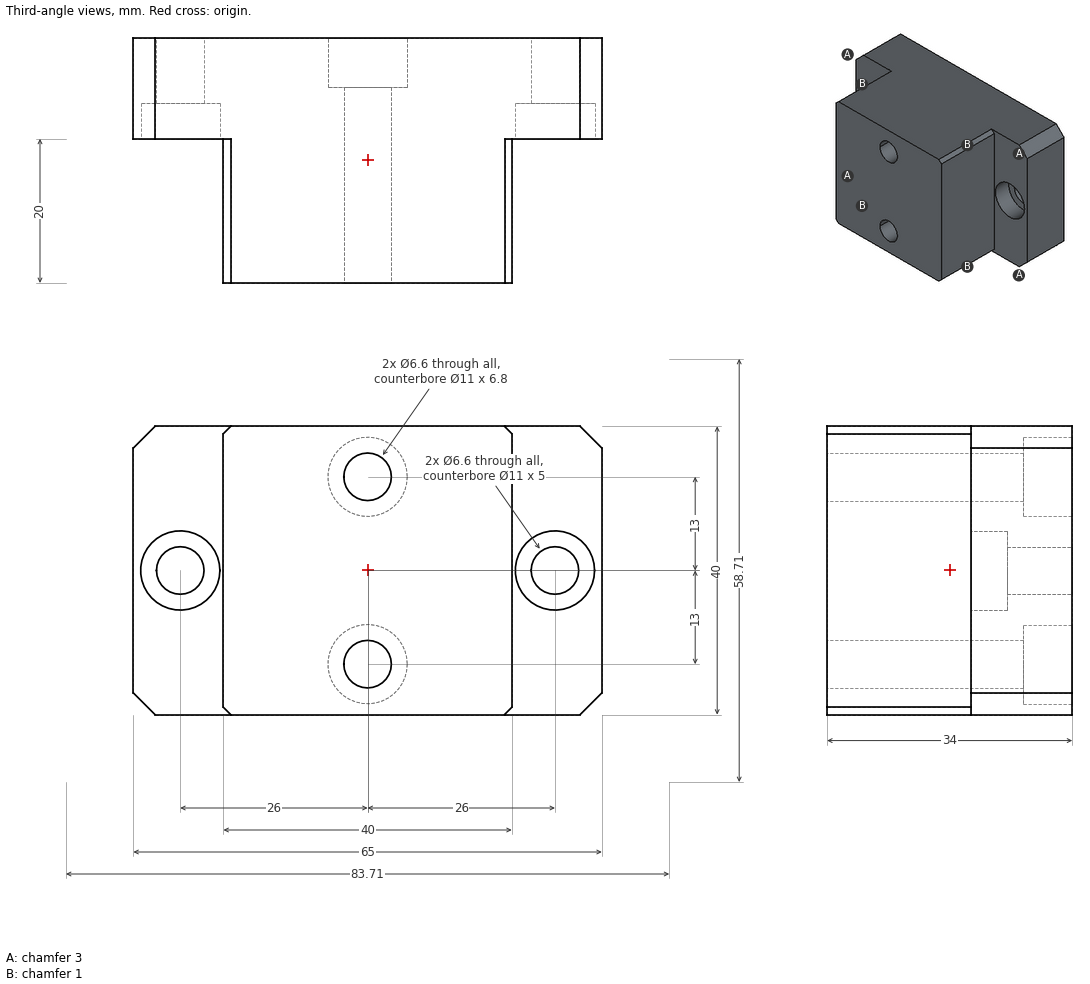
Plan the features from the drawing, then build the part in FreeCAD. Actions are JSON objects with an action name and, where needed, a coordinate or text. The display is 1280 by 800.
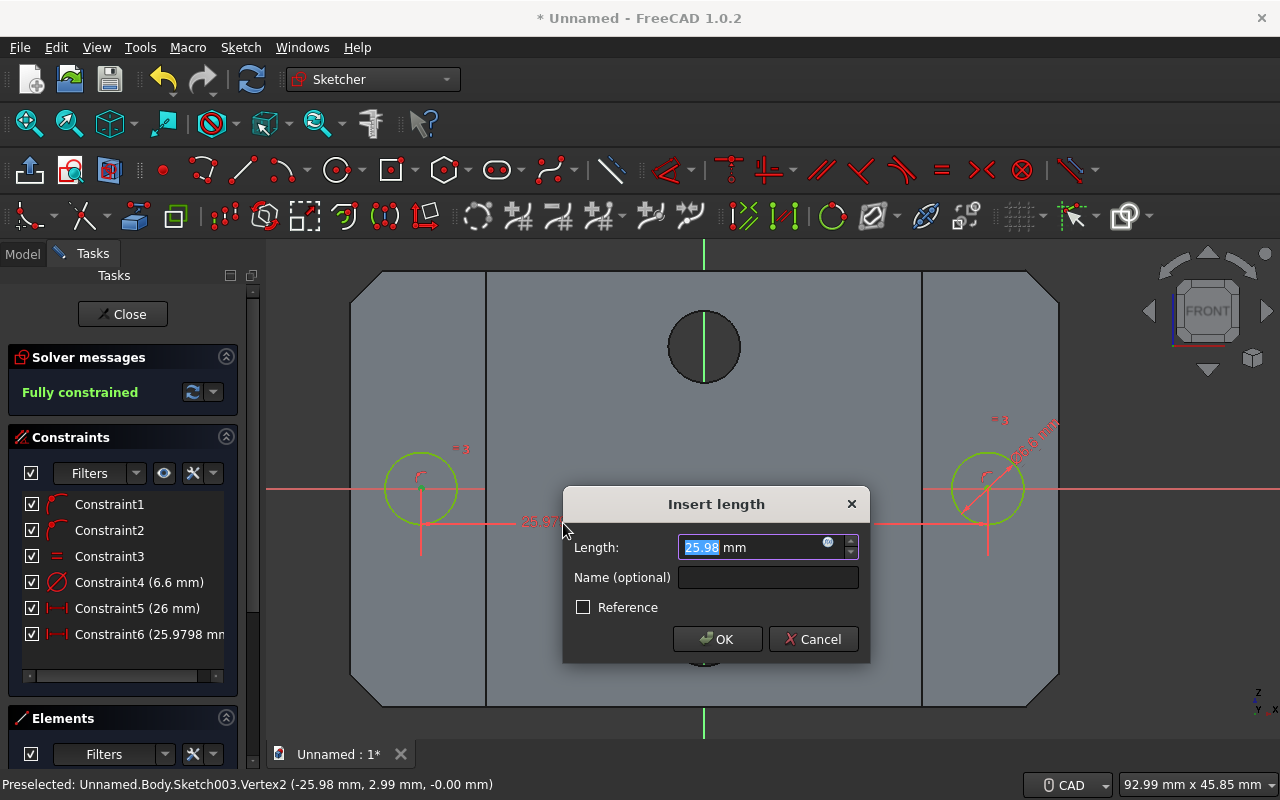
{"action": "type", "text": "26"}
{"action": "key", "text": "Return"}
{"action": "key", "text": "Escape"}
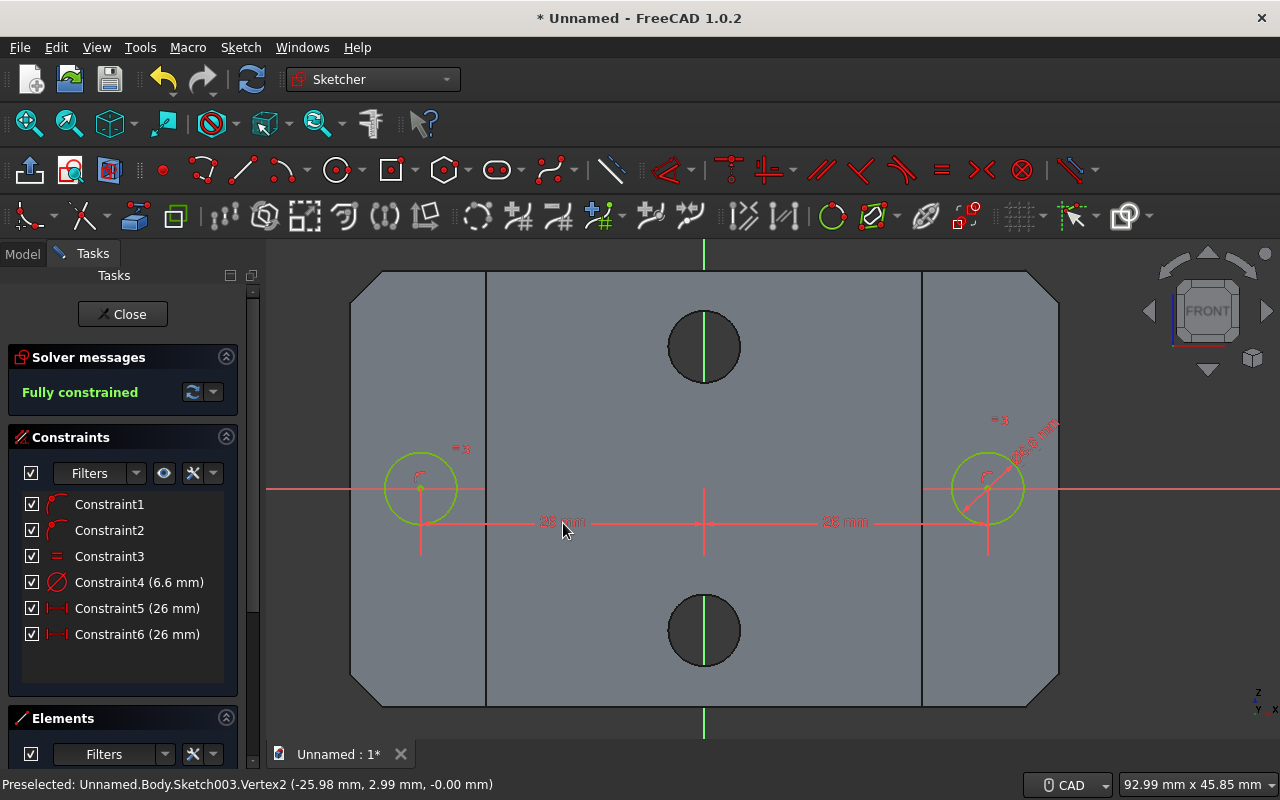
{"action": "left_click", "coordinate": [123, 314]}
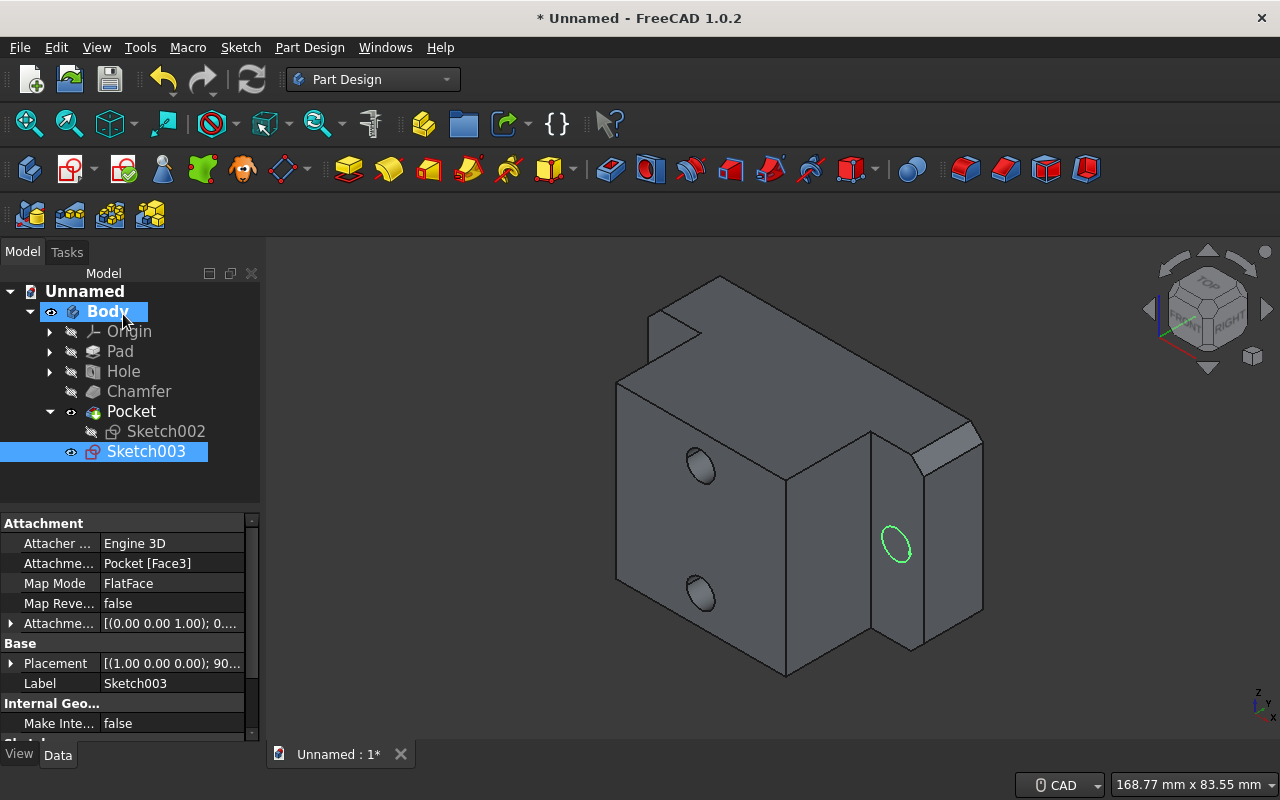
{"action": "left_click", "coordinate": [652, 170]}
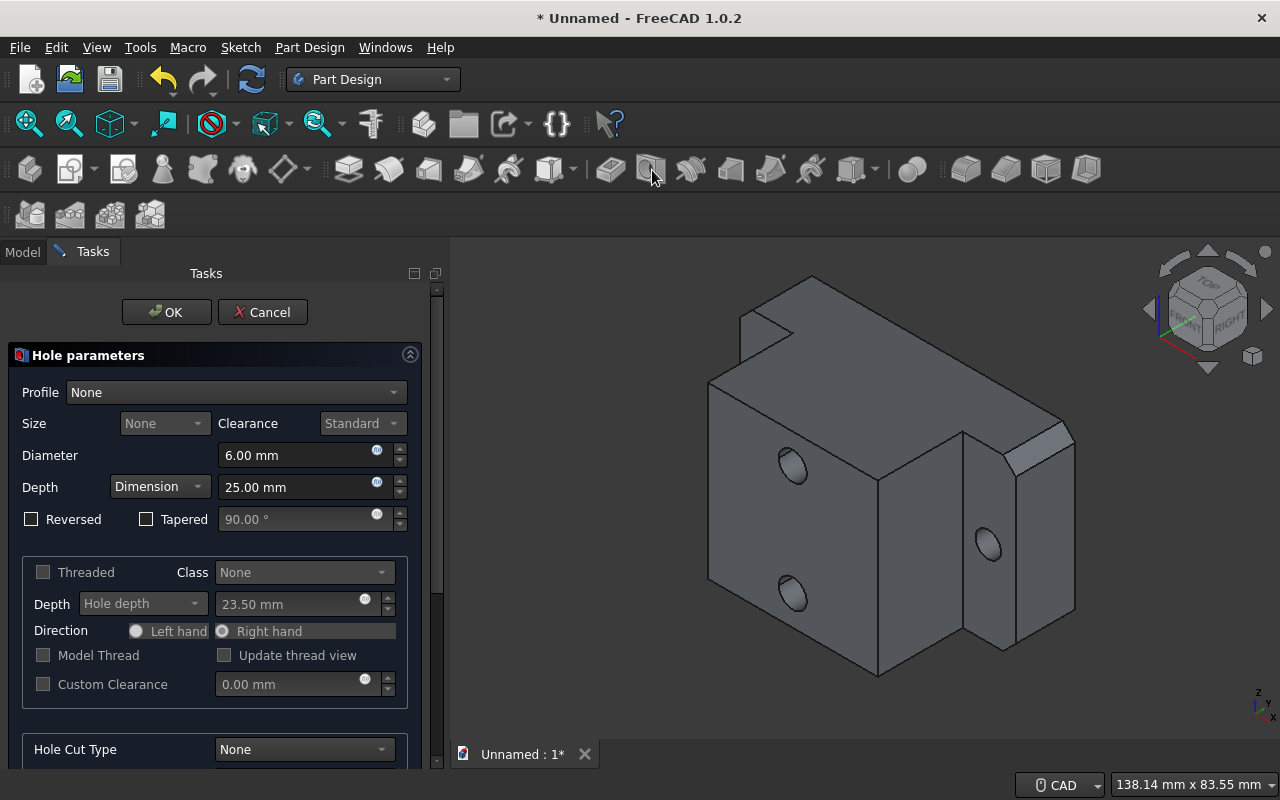
{"action": "triple_click", "coordinate": [305, 455]}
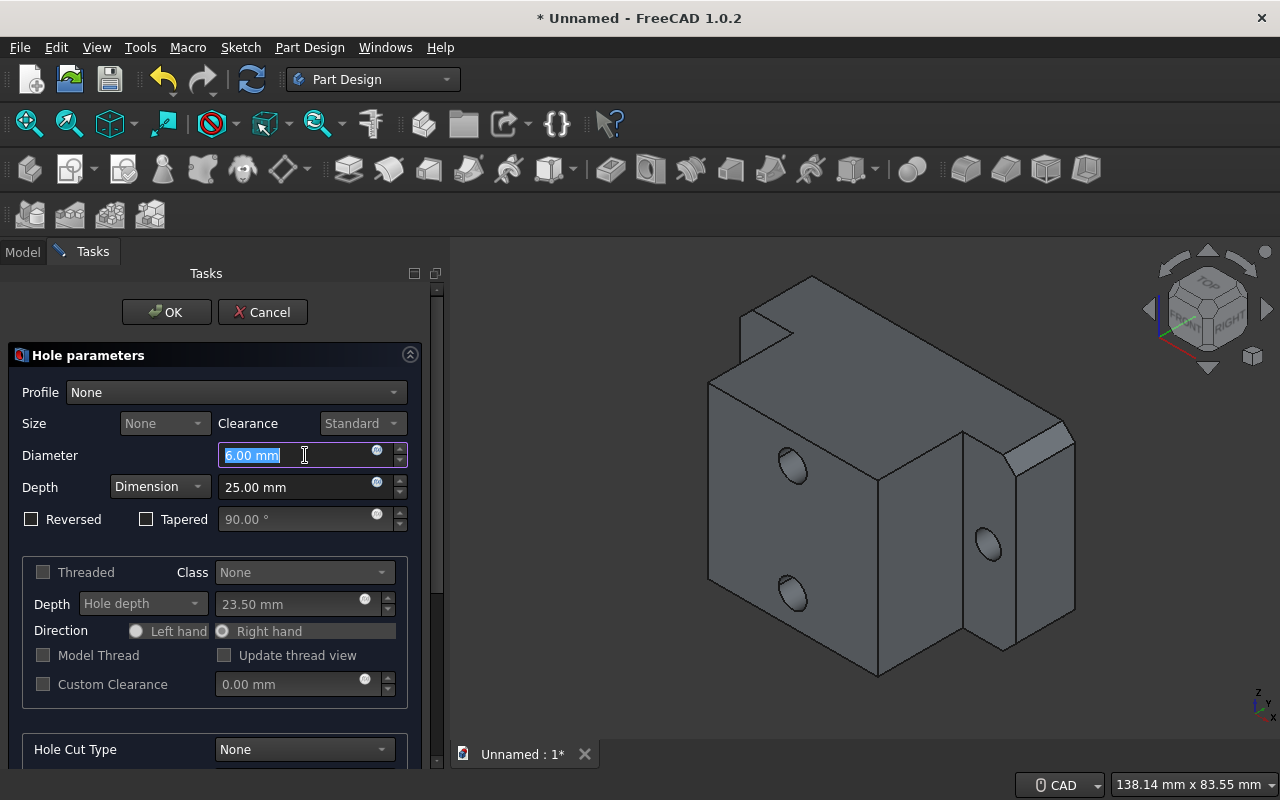
{"action": "type", "text": "6.6"}
{"action": "key", "text": "Tab"}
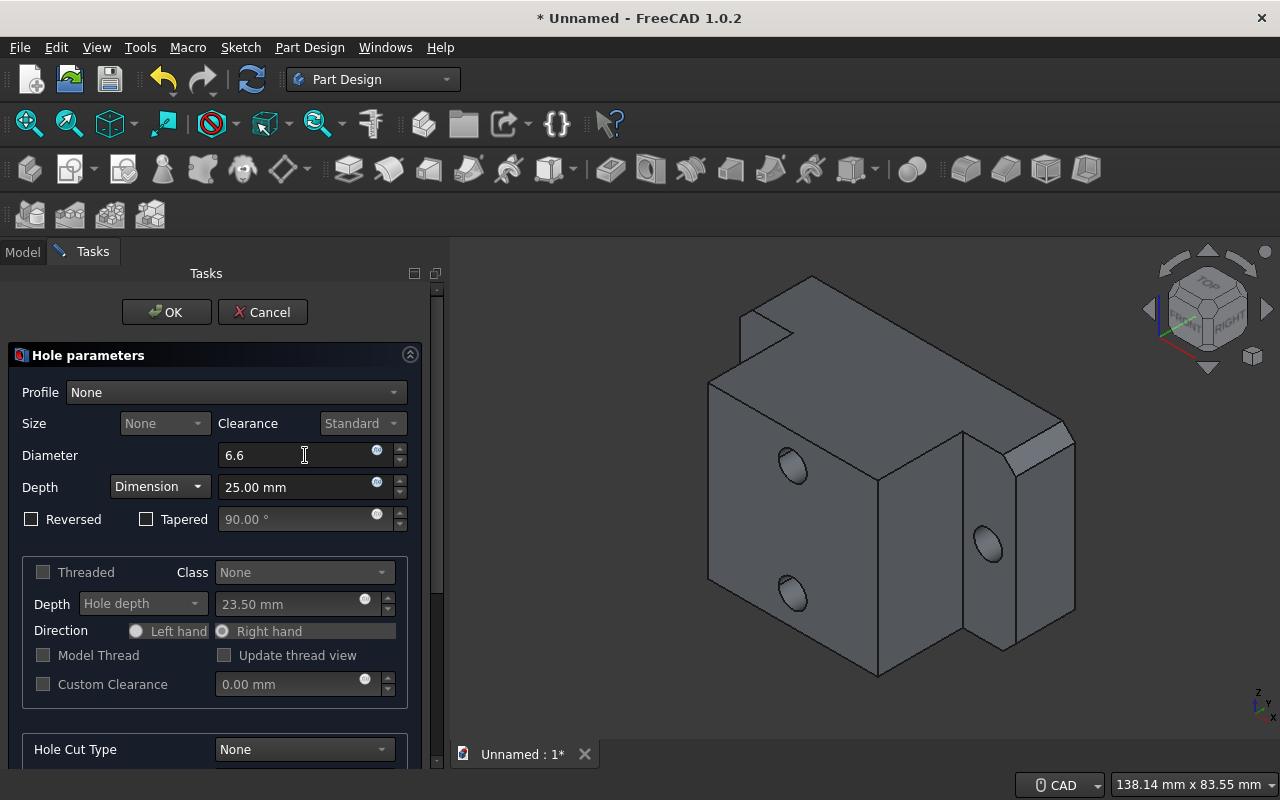
{"action": "left_click", "coordinate": [161, 486]}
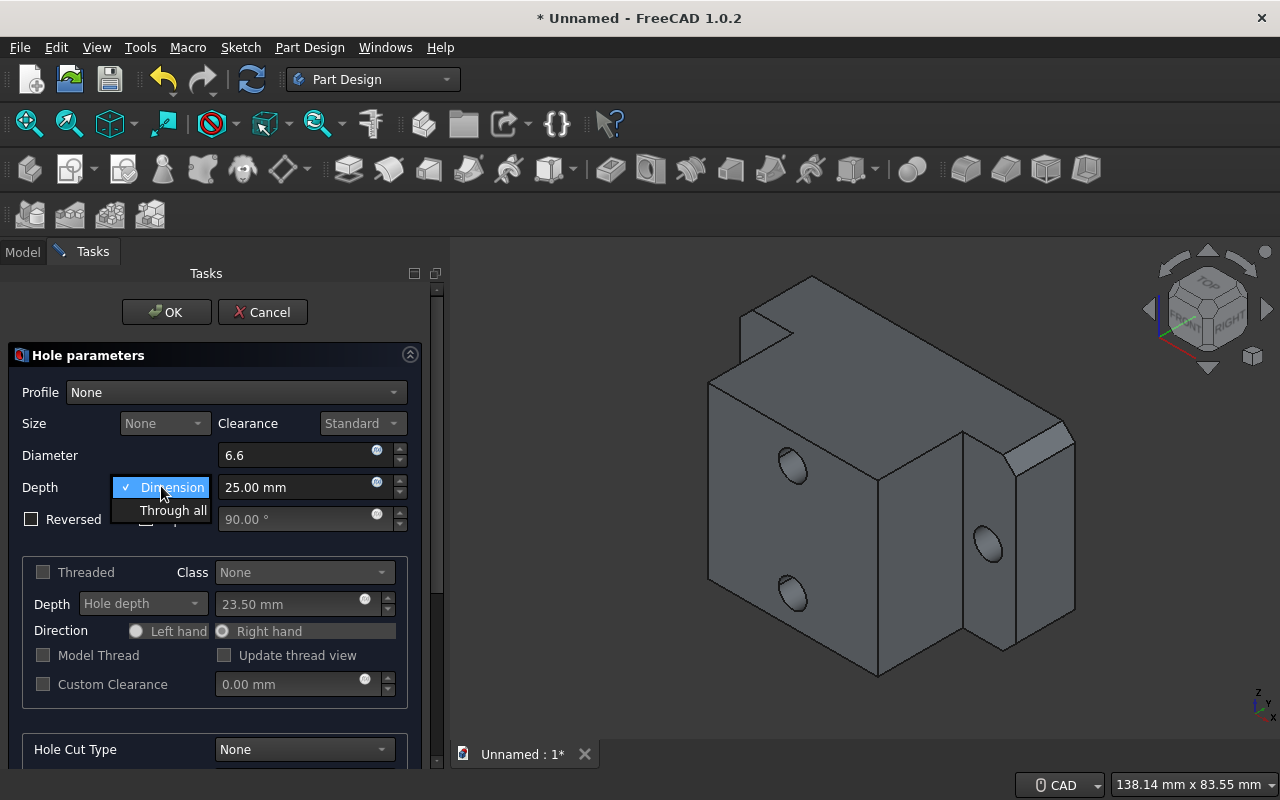
{"action": "left_click", "coordinate": [160, 510]}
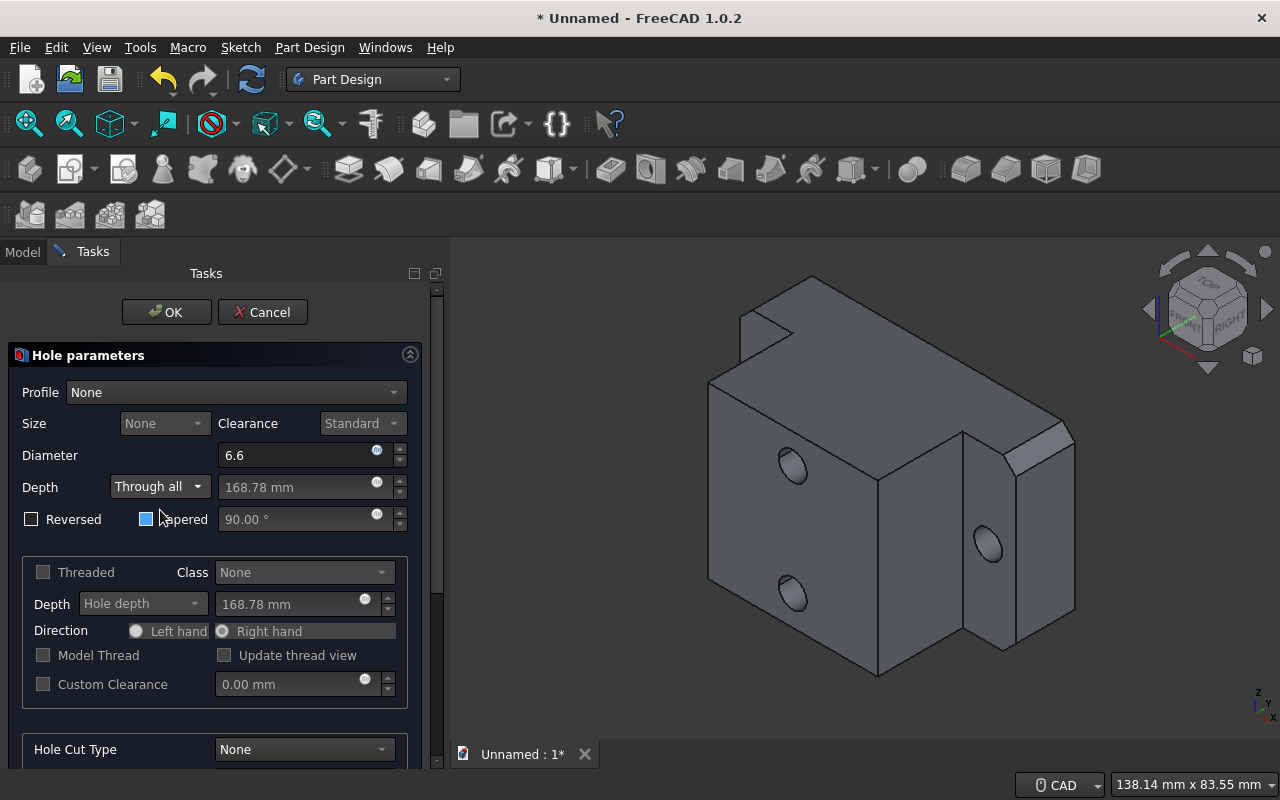
{"action": "left_click", "coordinate": [306, 750]}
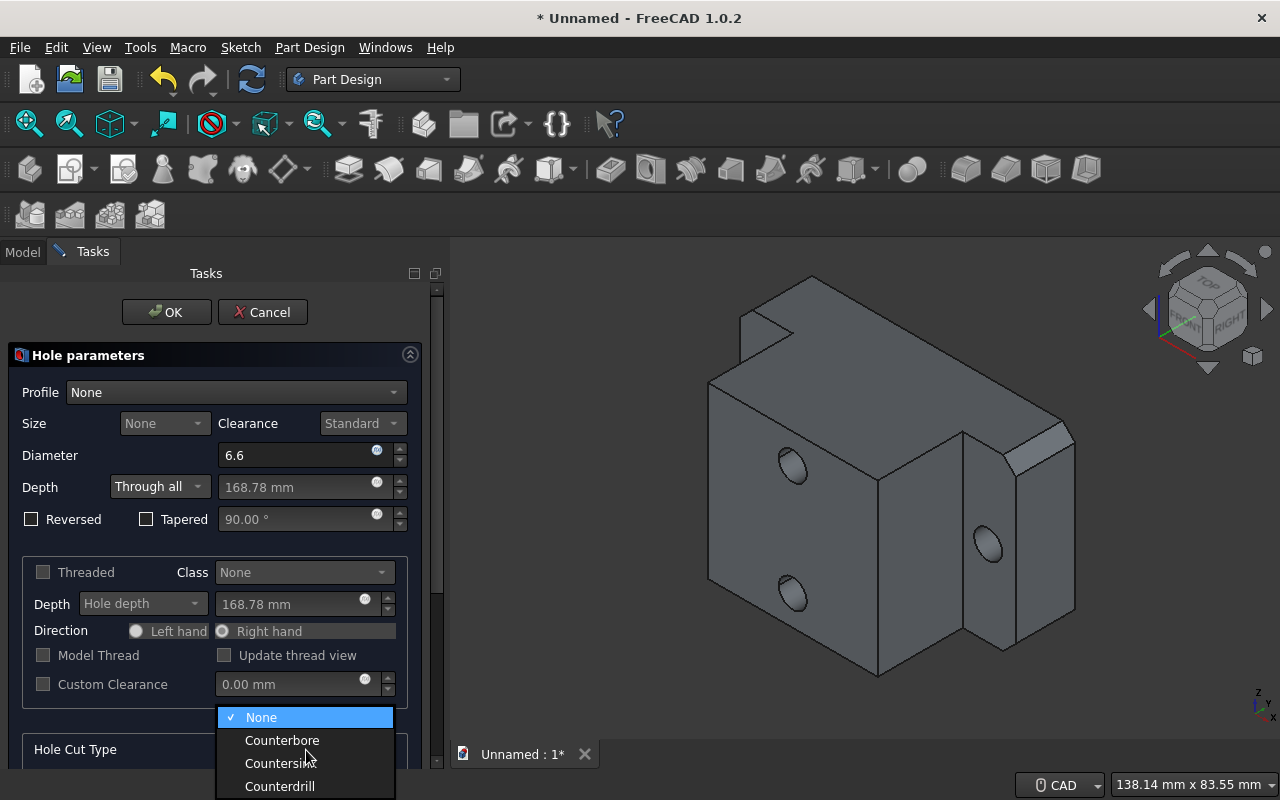
{"action": "left_click", "coordinate": [304, 740]}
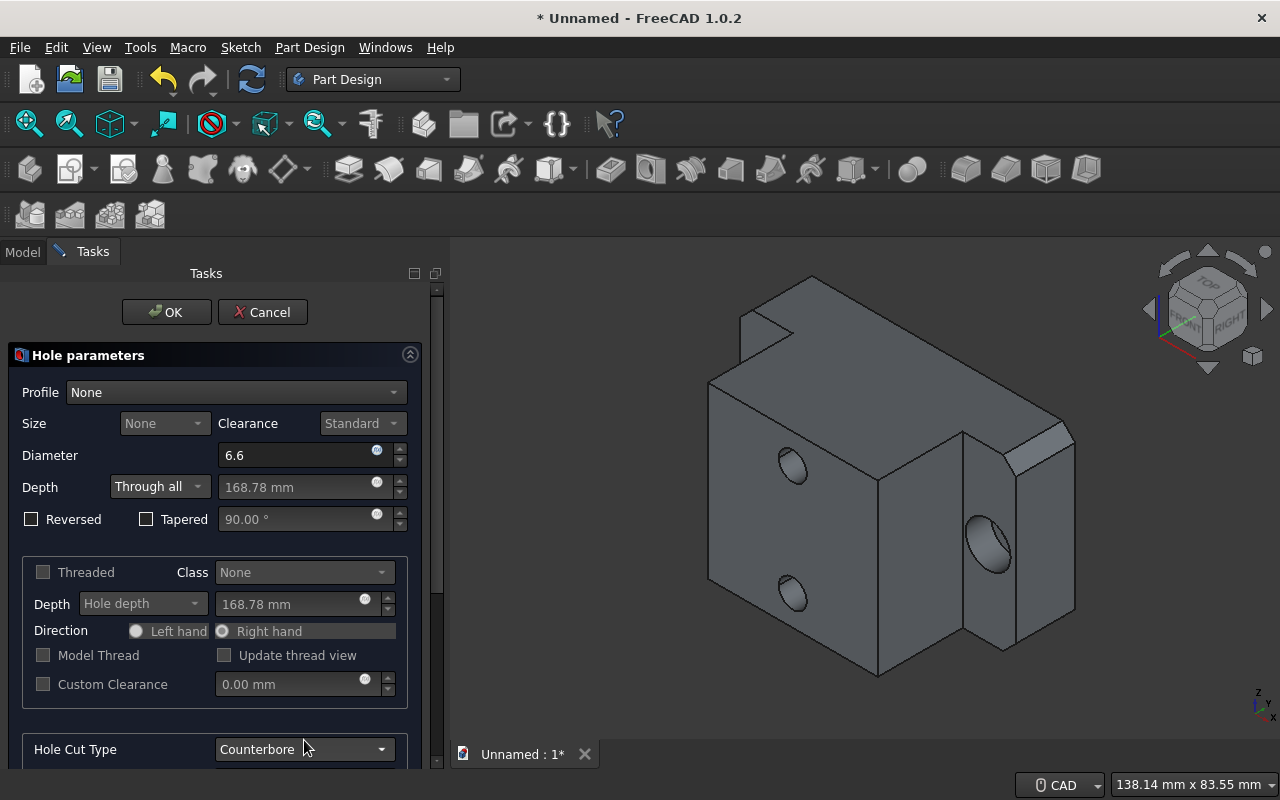
{"action": "scroll", "coordinate": [437, 526], "scroll_direction": "down", "scroll_amount": 2}